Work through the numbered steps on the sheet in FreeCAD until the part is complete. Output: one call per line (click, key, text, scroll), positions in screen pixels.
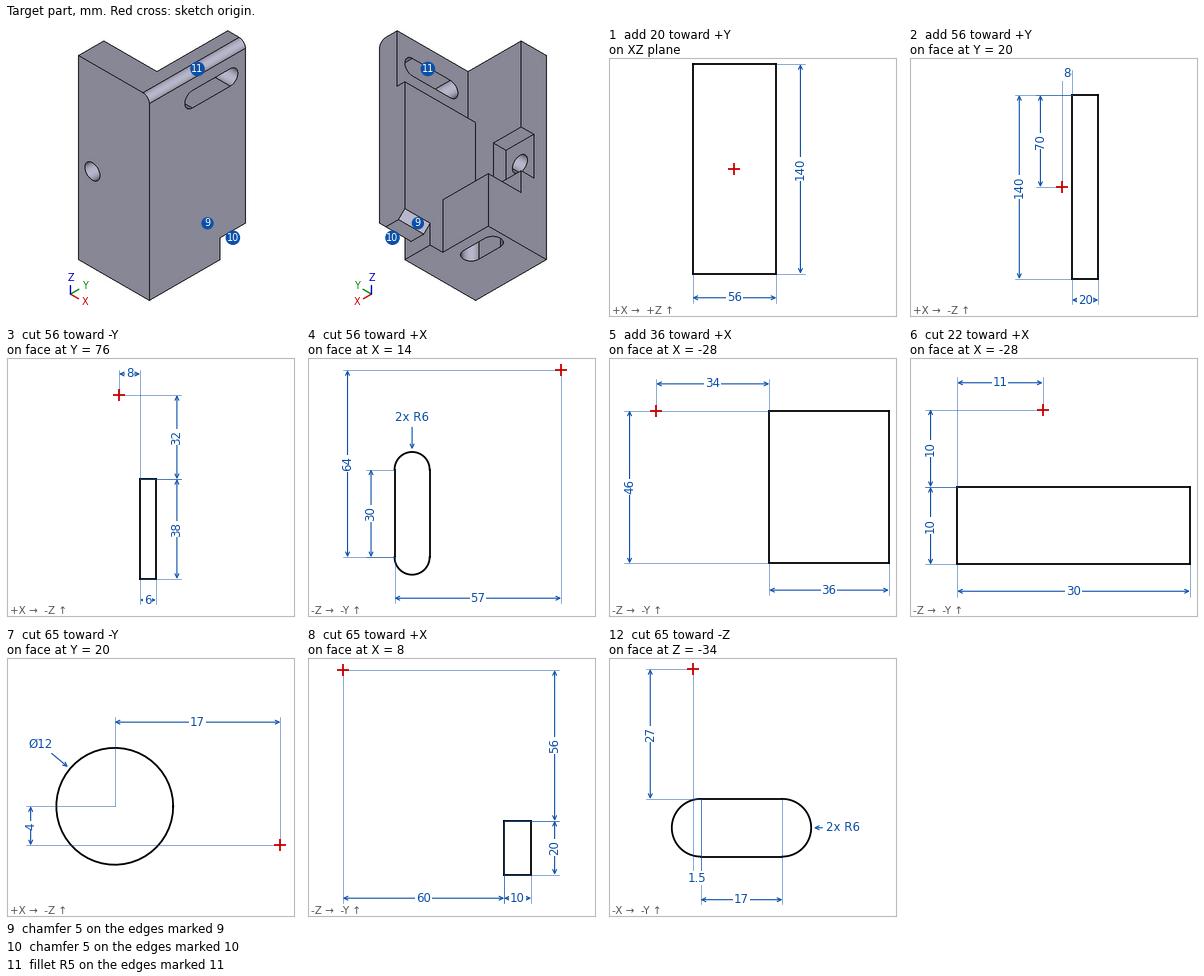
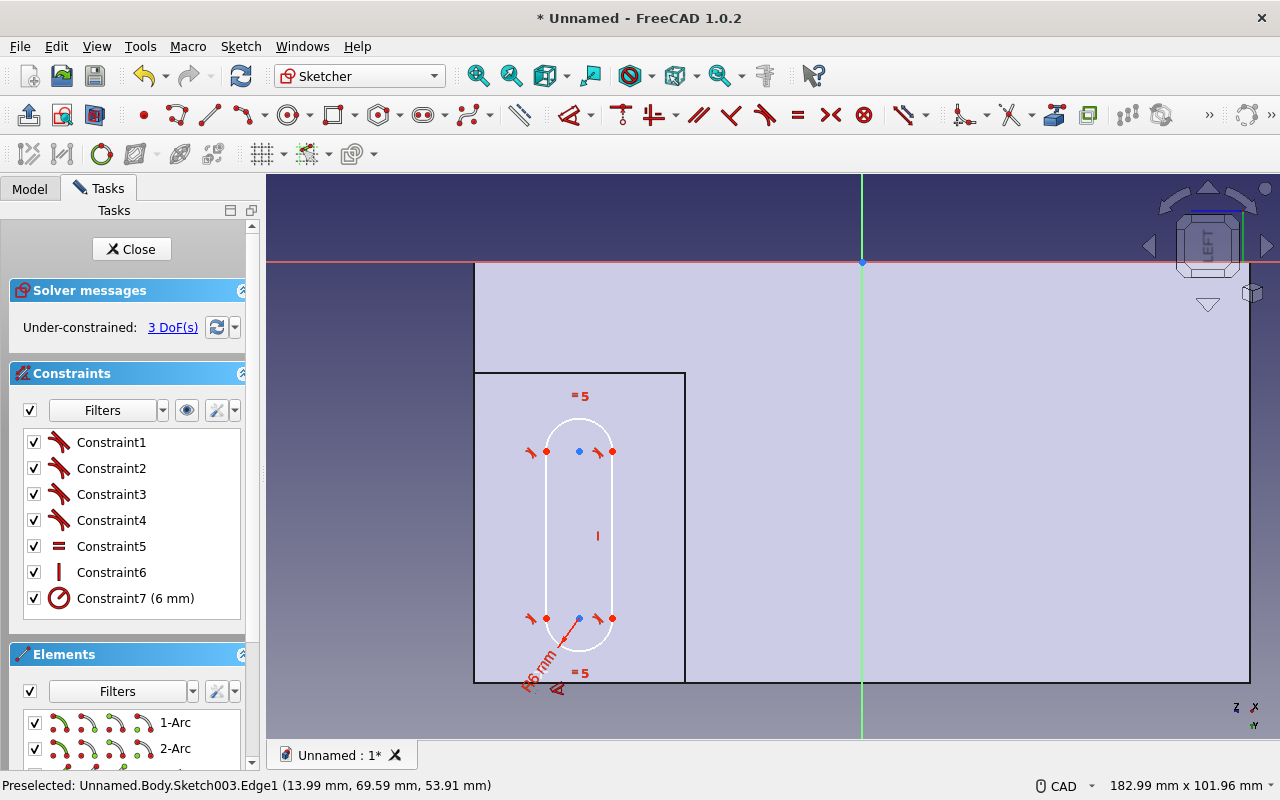
click(546, 568)
click(512, 535)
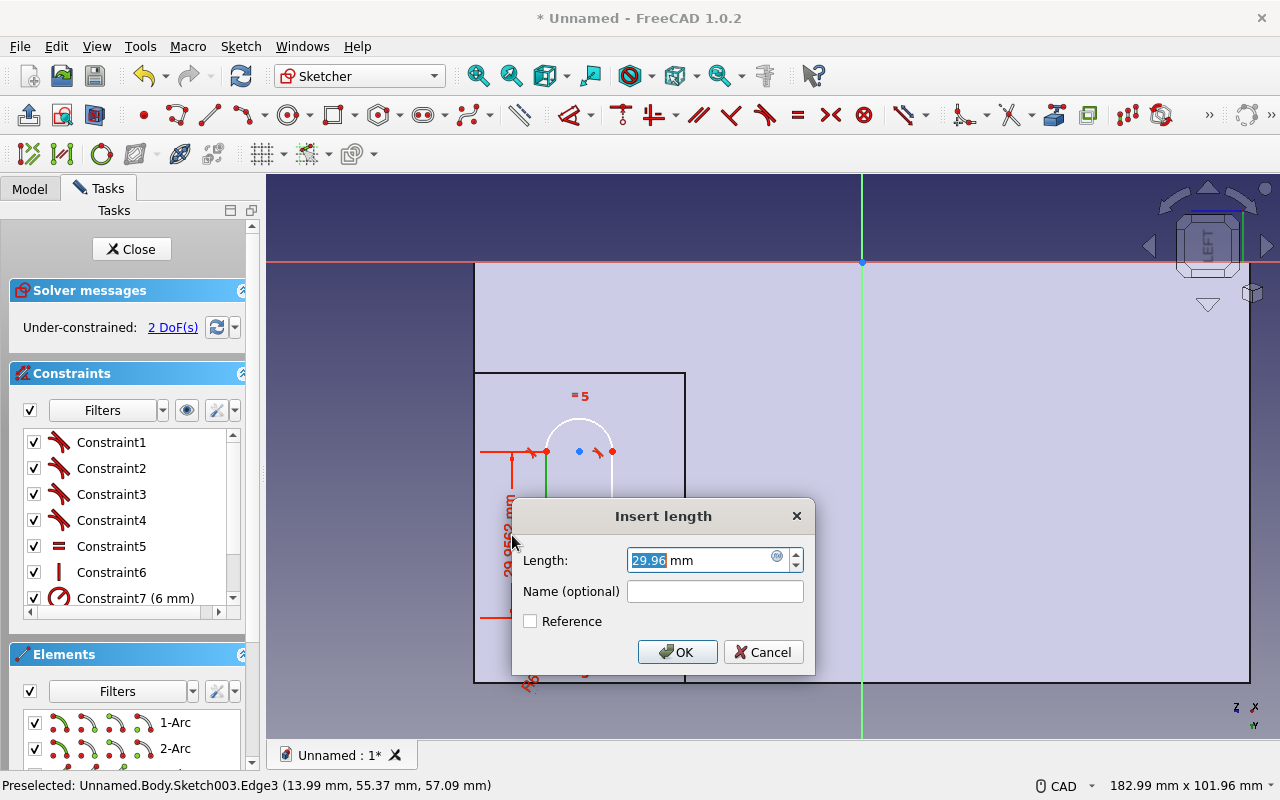
text(30)
key(Return)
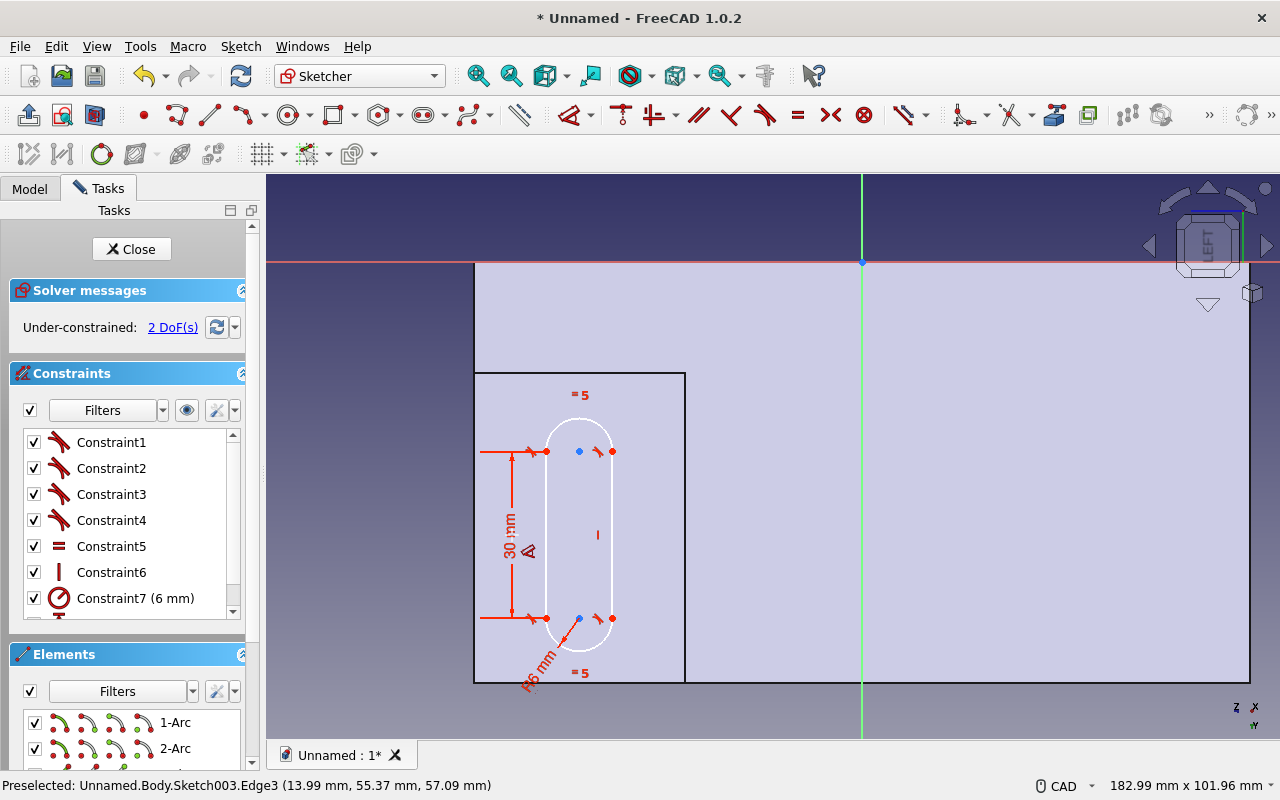
click(546, 618)
click(704, 228)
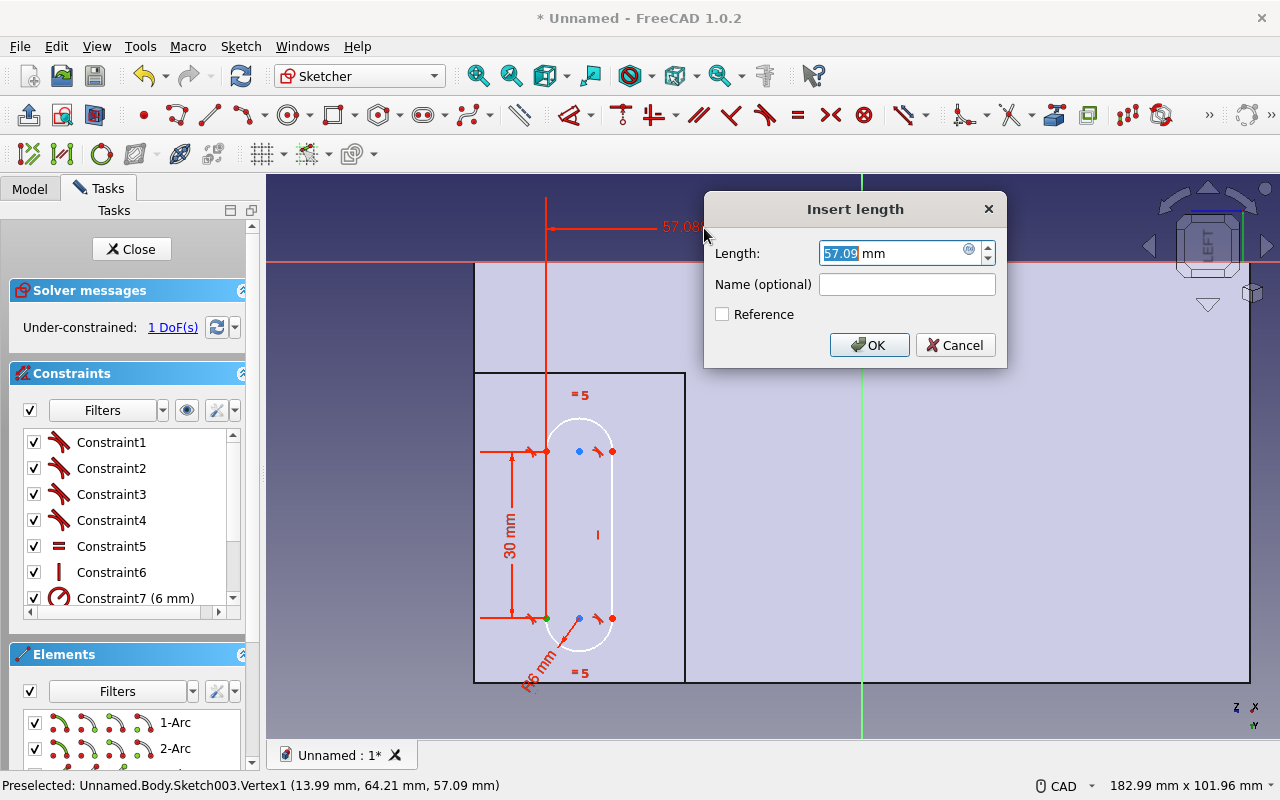
text(57)
key(Return)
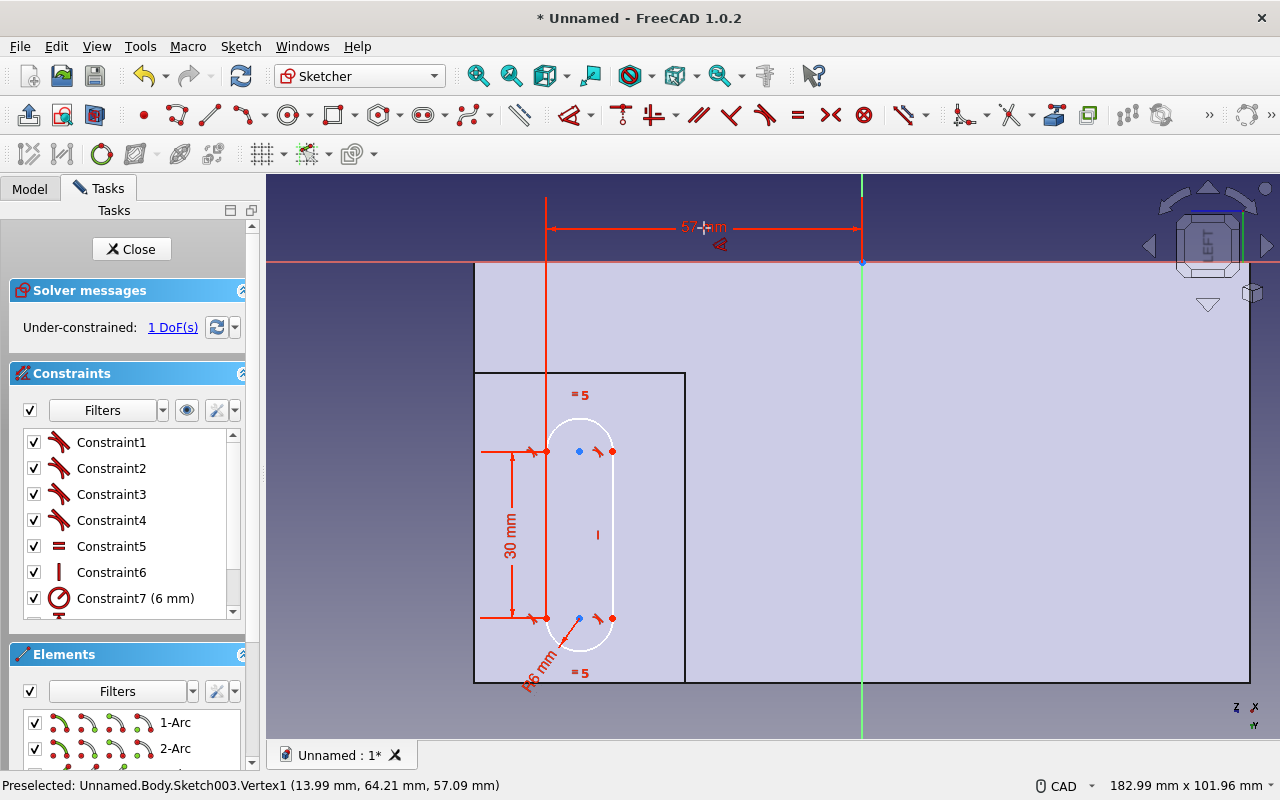
click(546, 618)
click(896, 440)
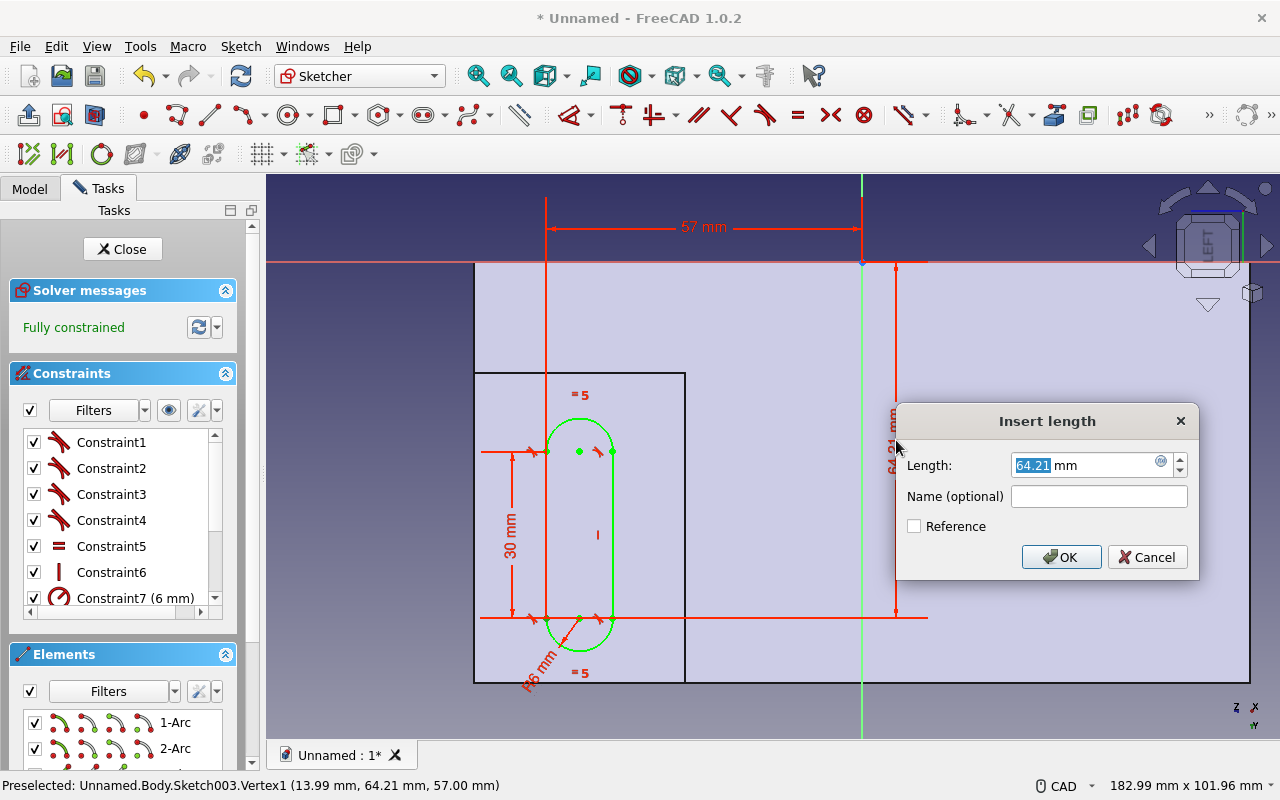
text(64)
key(Return)
key(Escape)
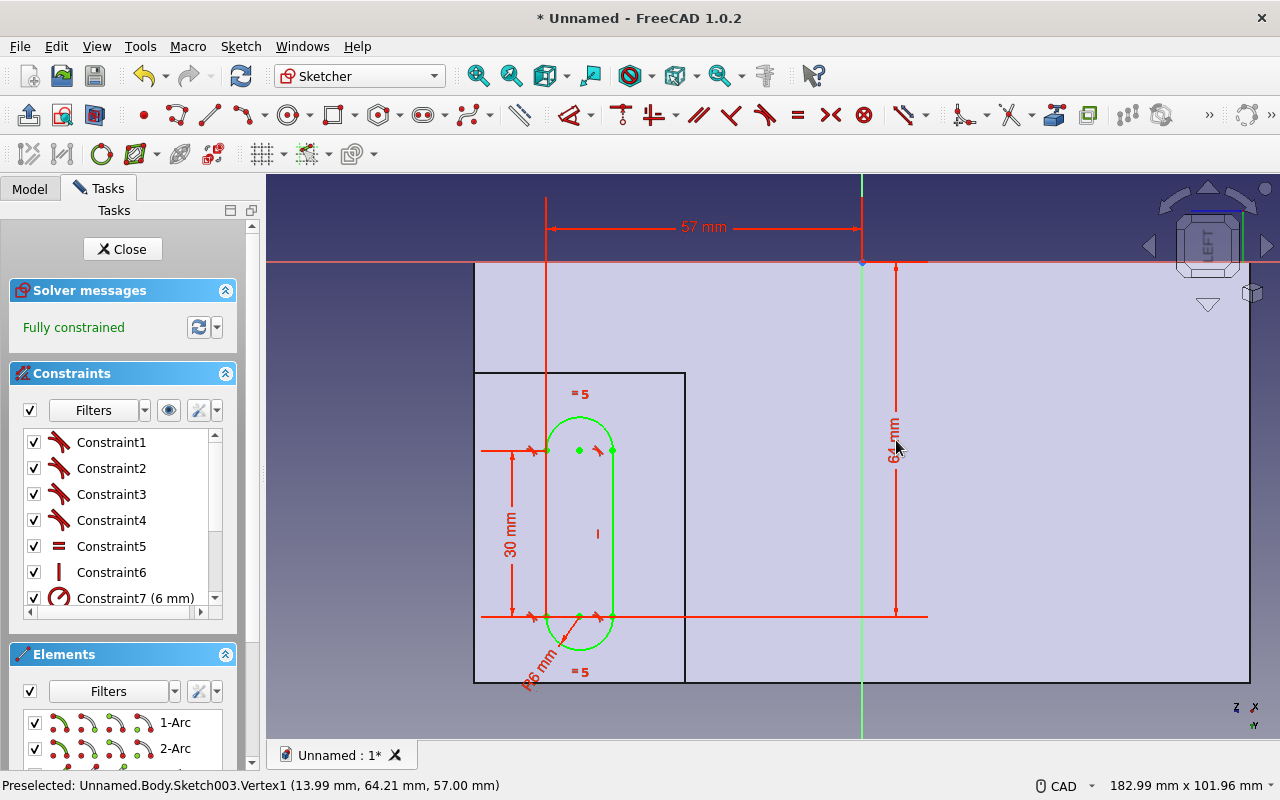
click(123, 249)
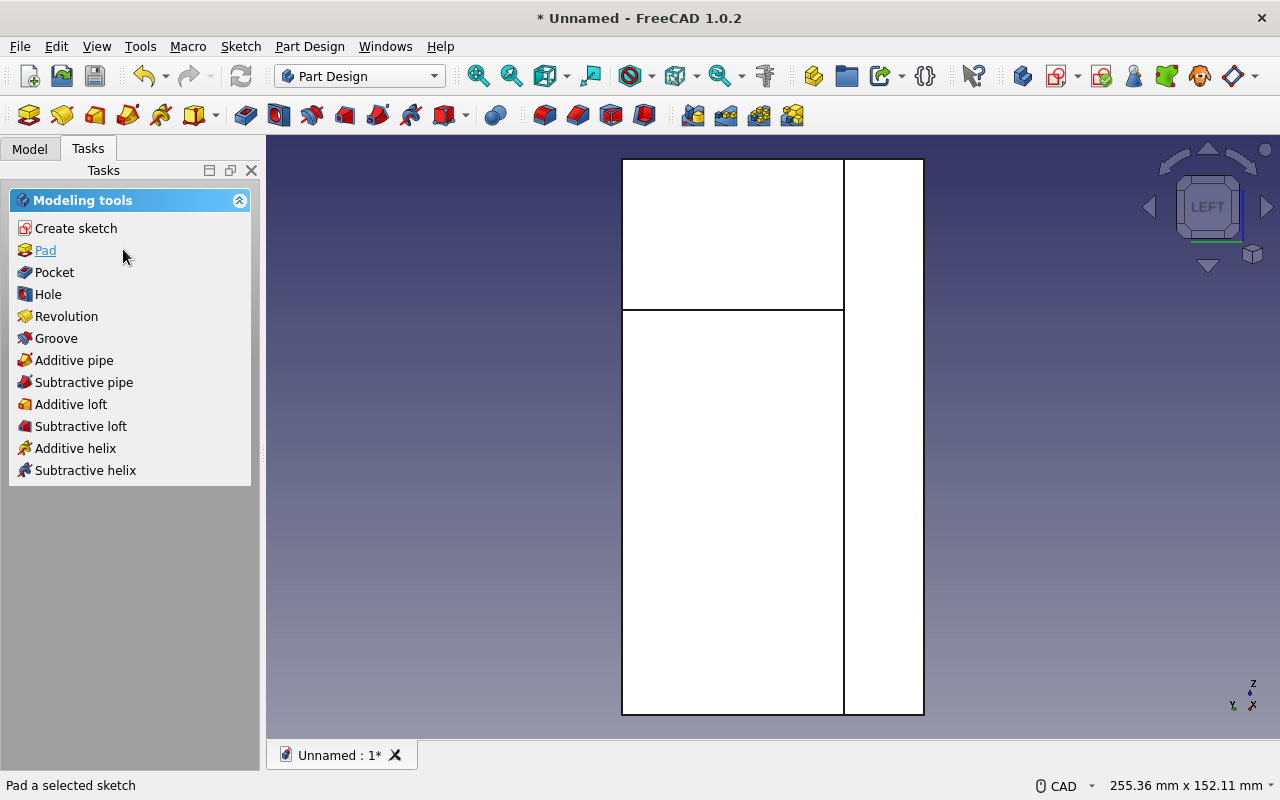
click(246, 116)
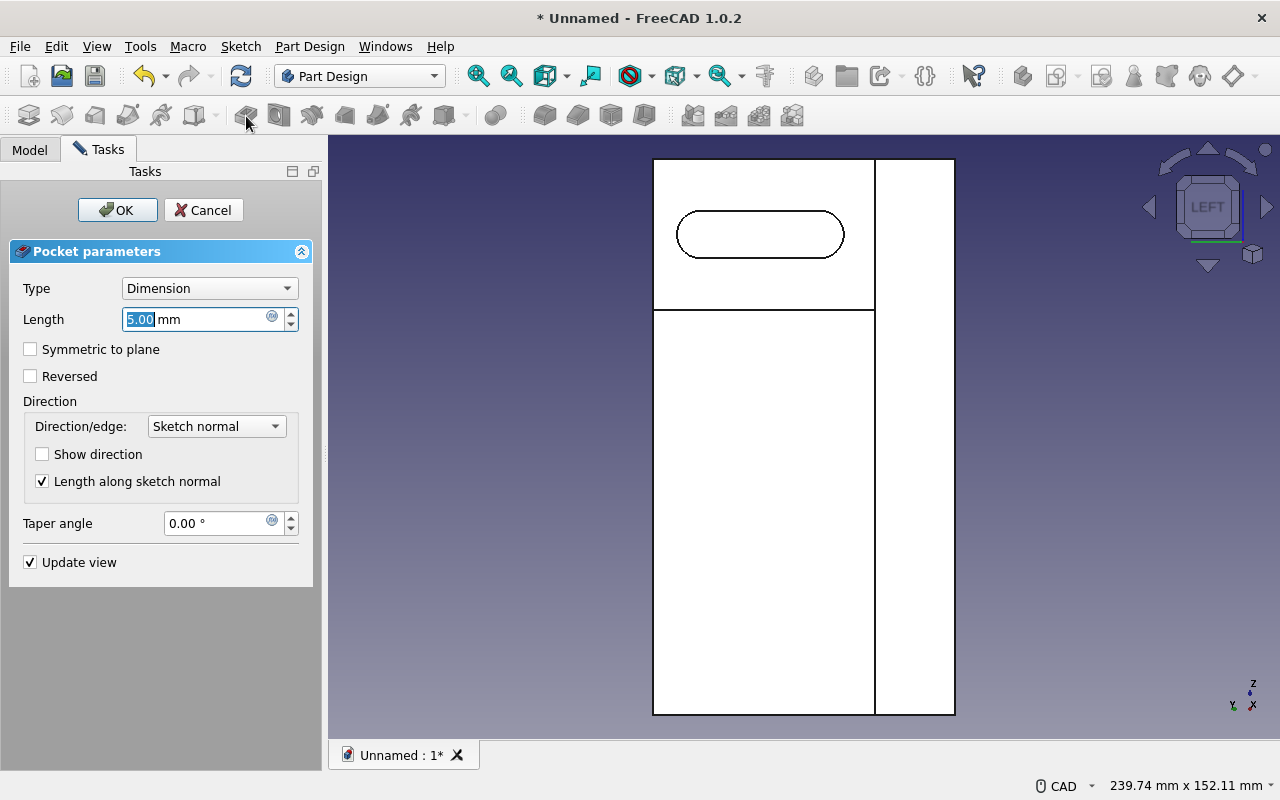
text(56)
key(Tab)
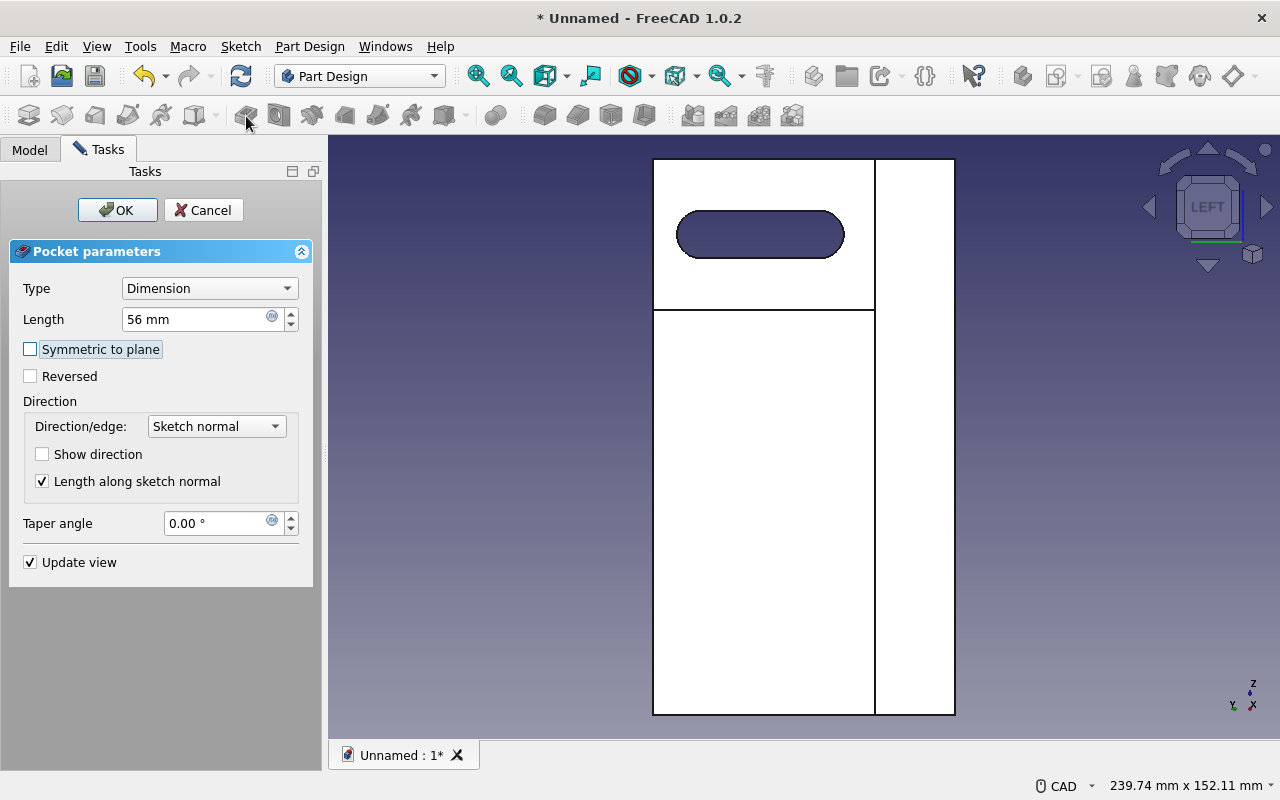
click(118, 210)